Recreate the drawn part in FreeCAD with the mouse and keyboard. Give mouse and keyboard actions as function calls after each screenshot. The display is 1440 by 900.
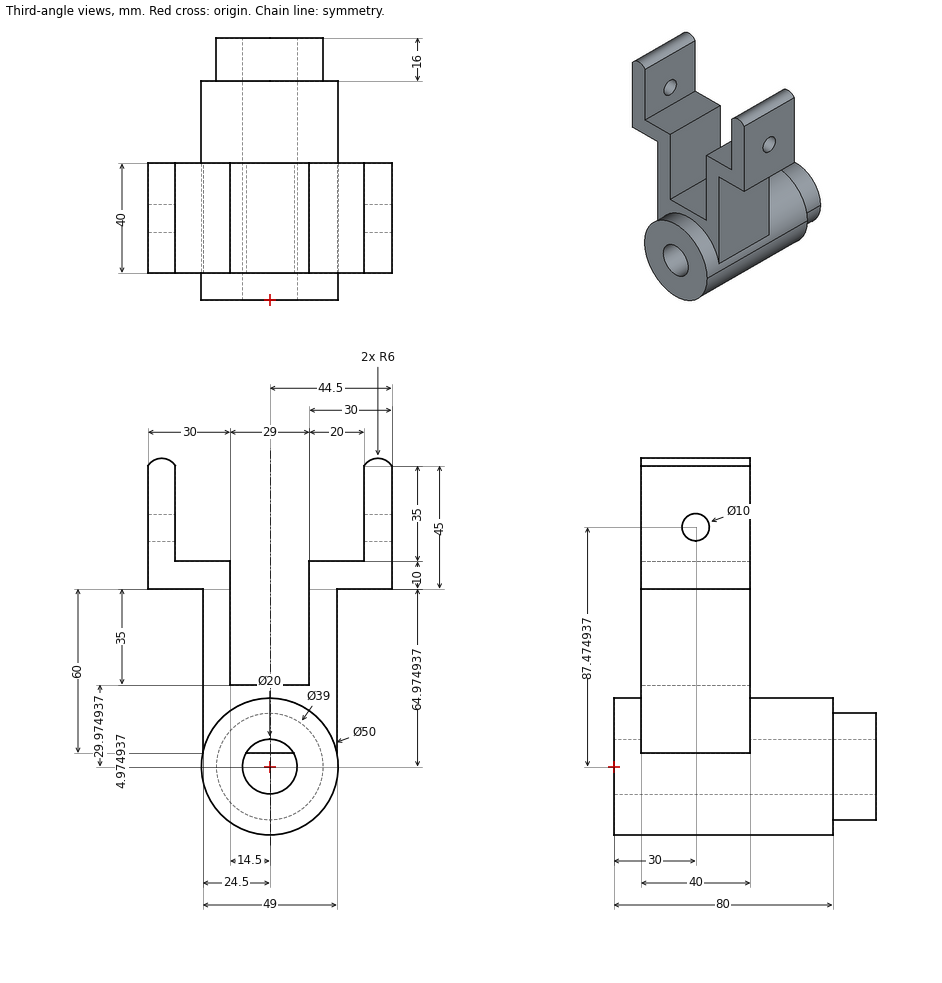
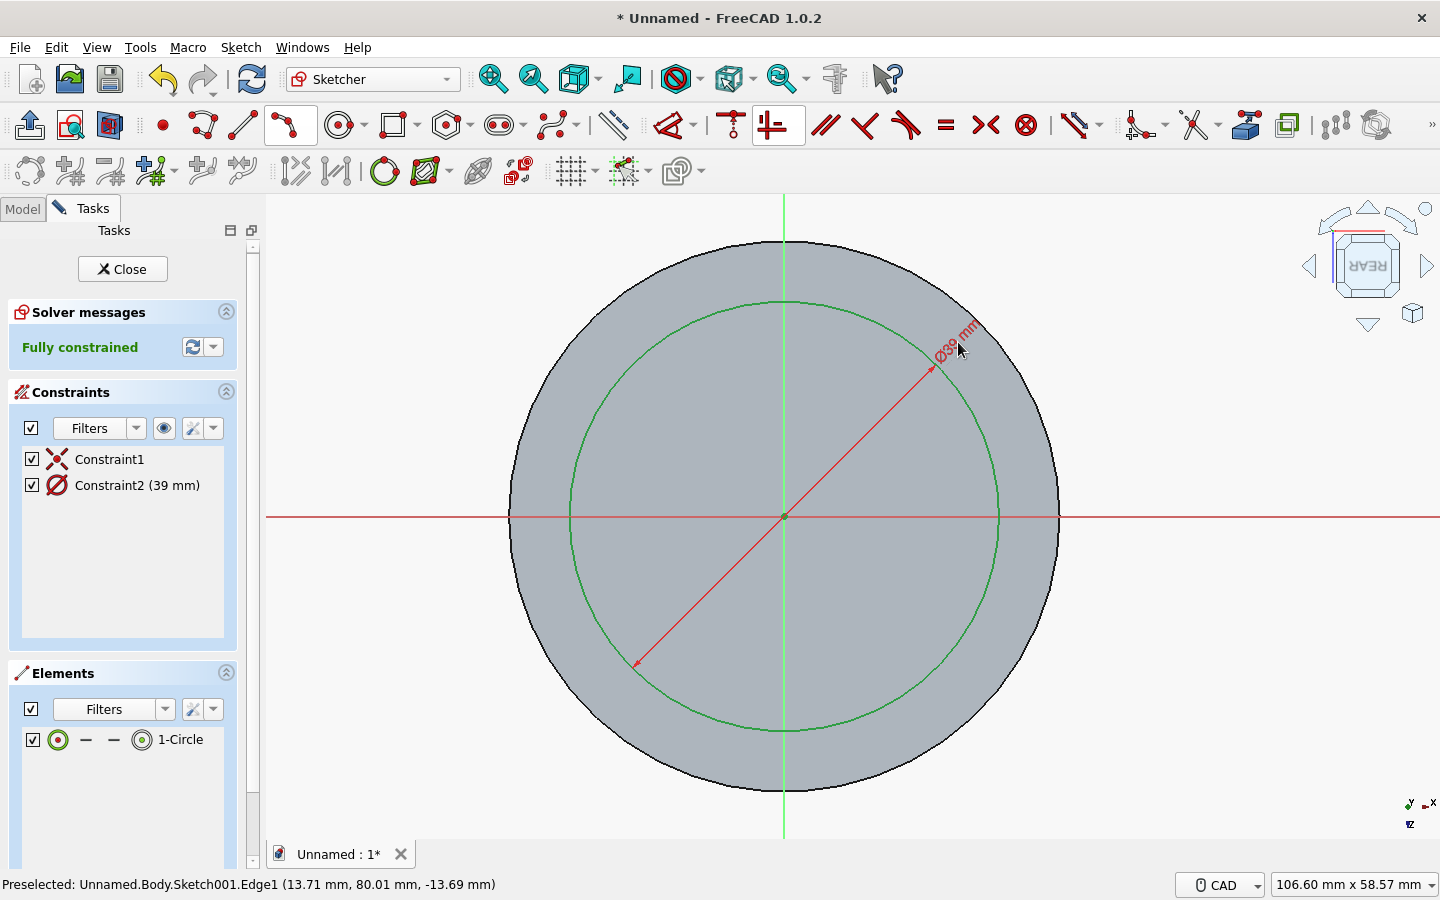
click(123, 269)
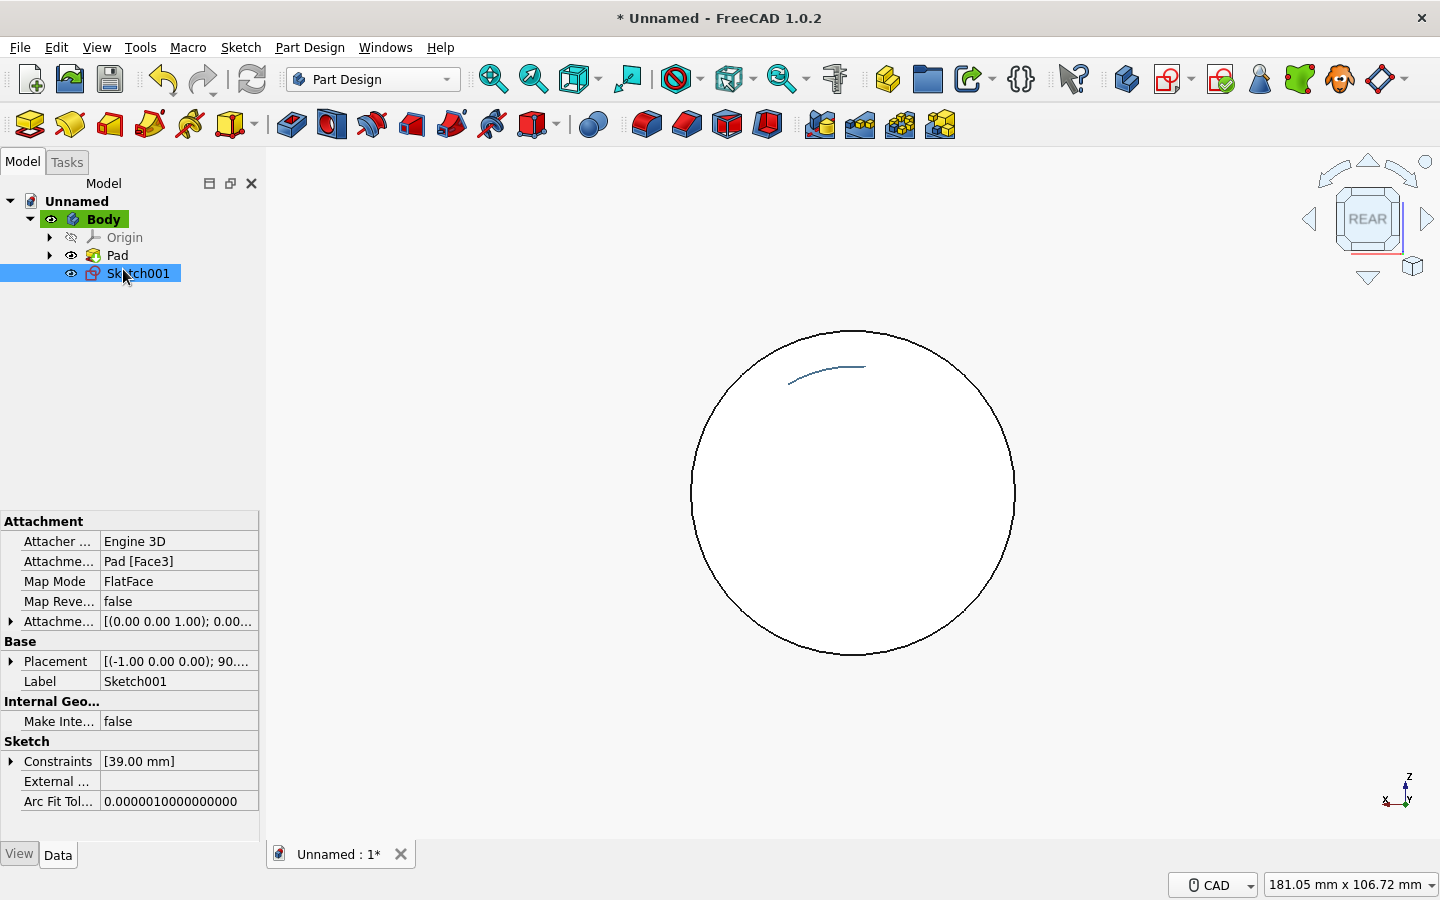
click(30, 124)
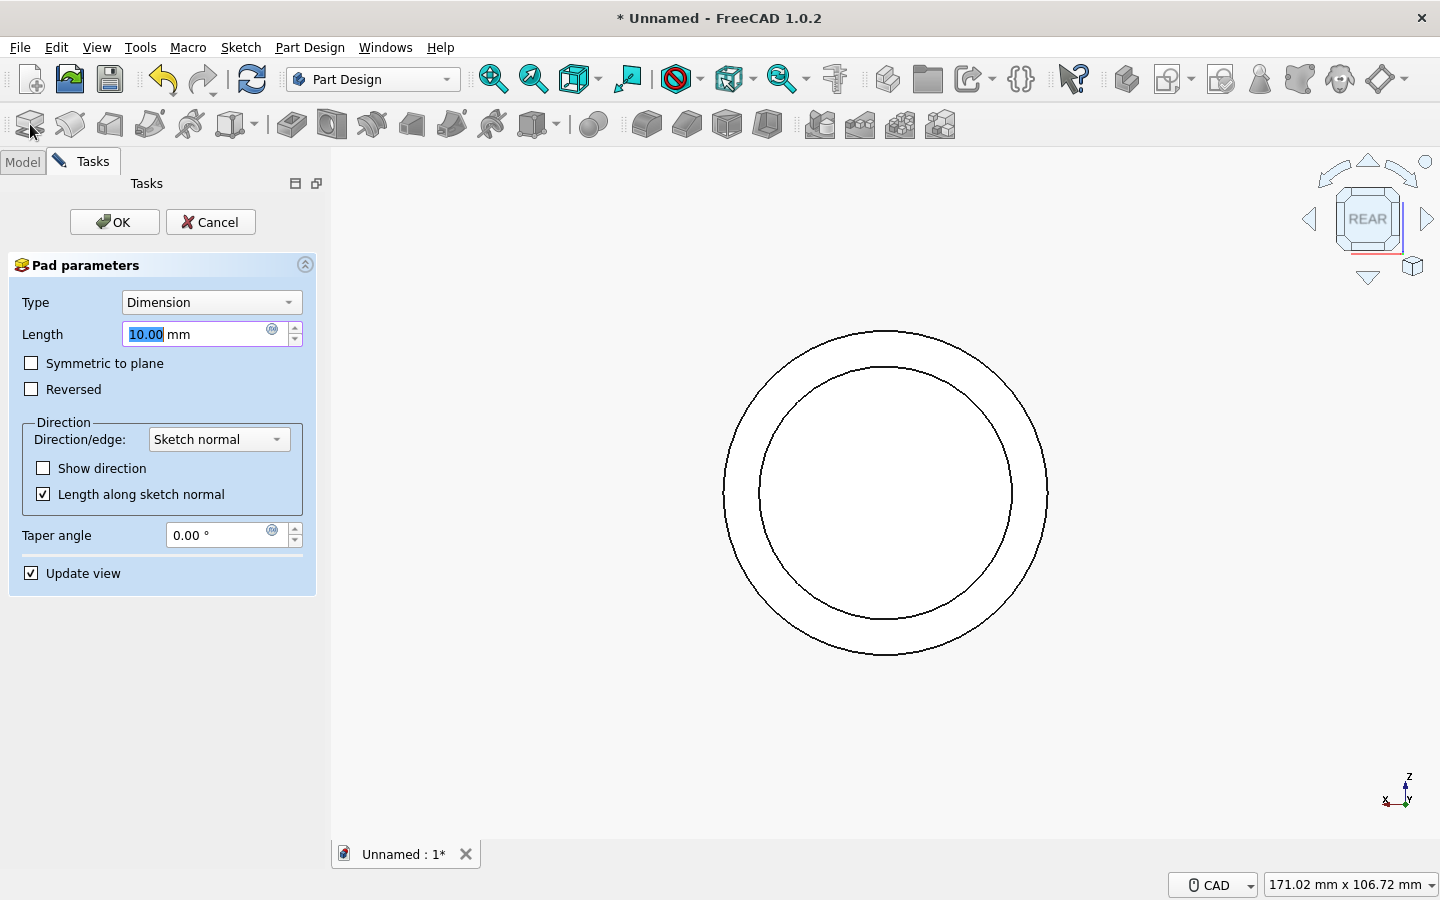
text(16)
key(Tab)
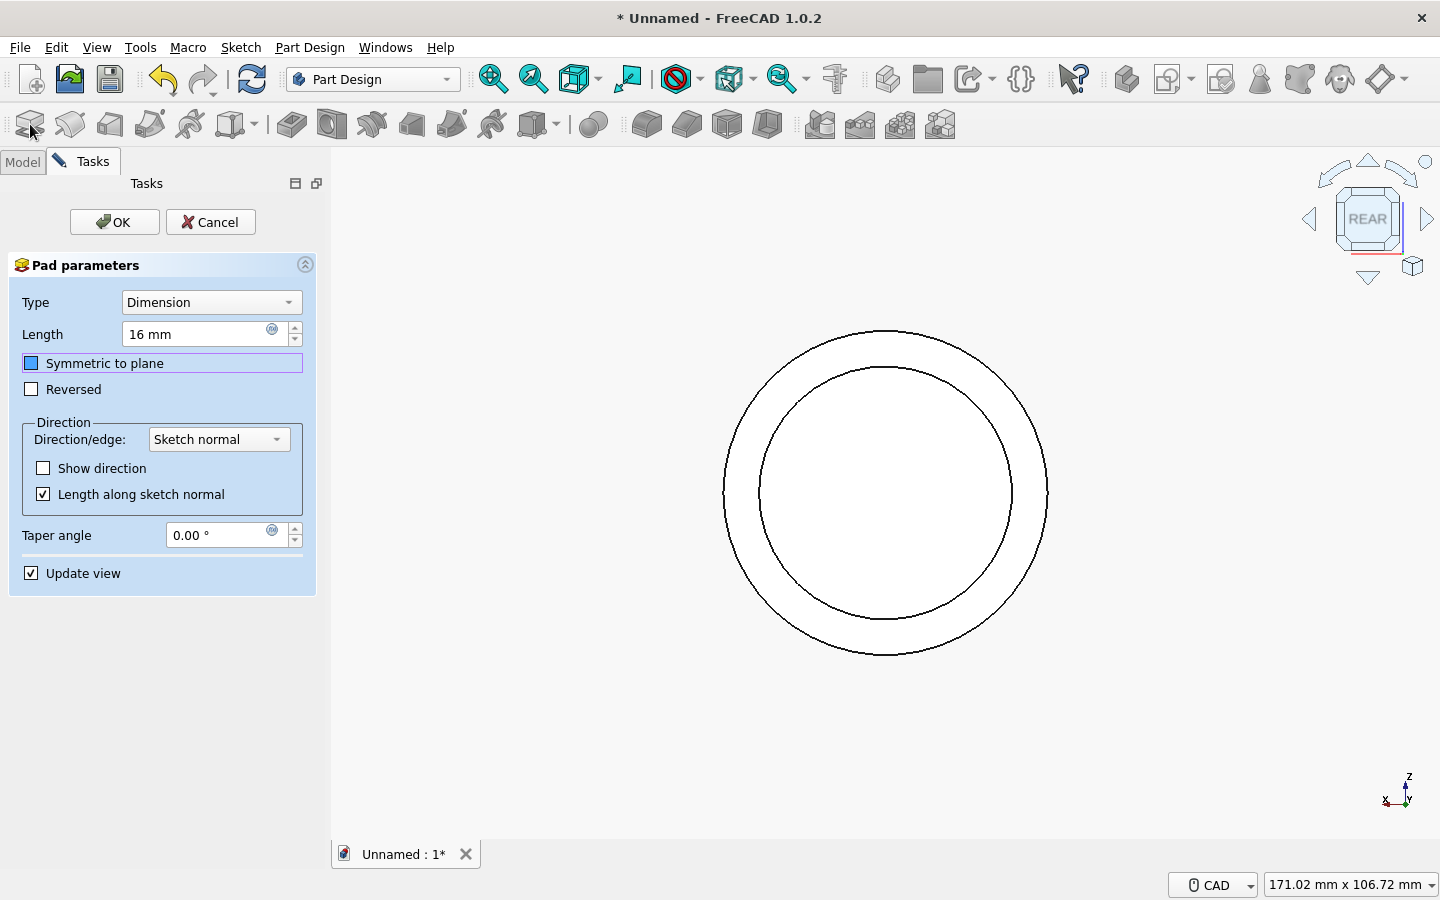
click(115, 222)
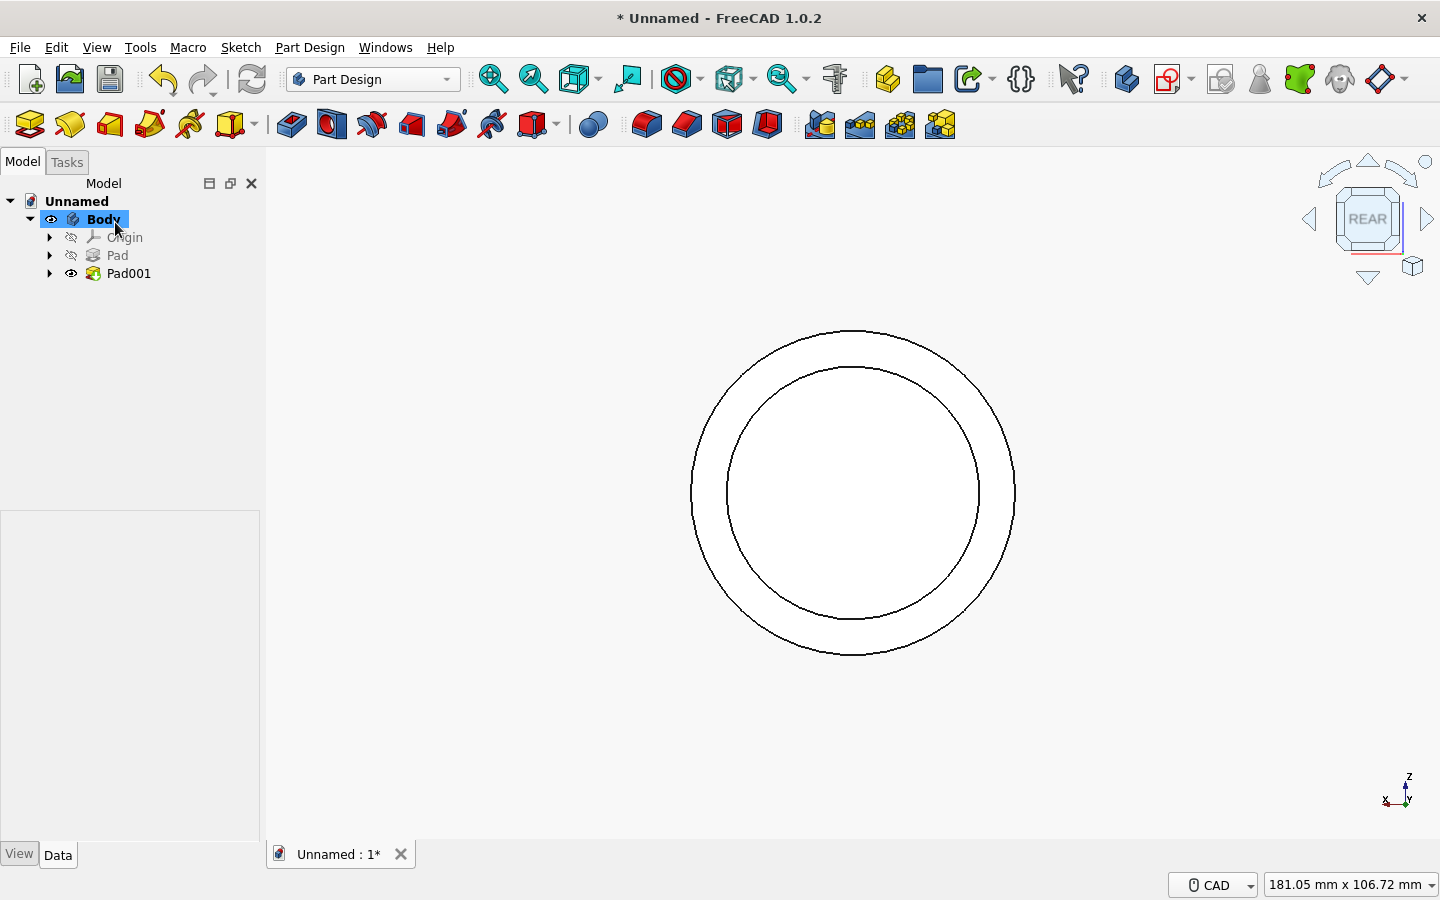
click(853, 492)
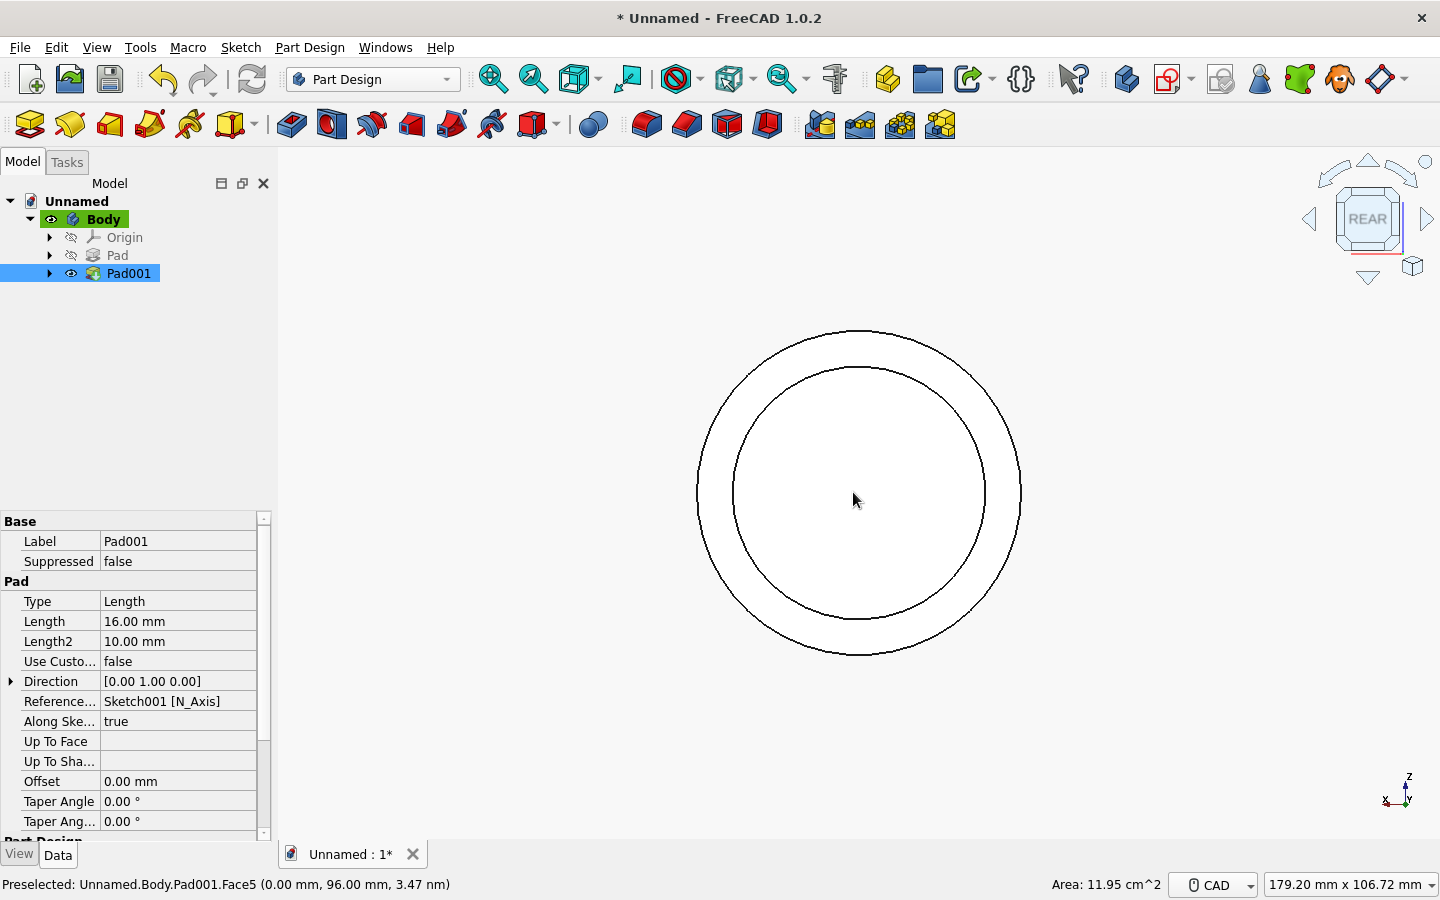
click(1168, 80)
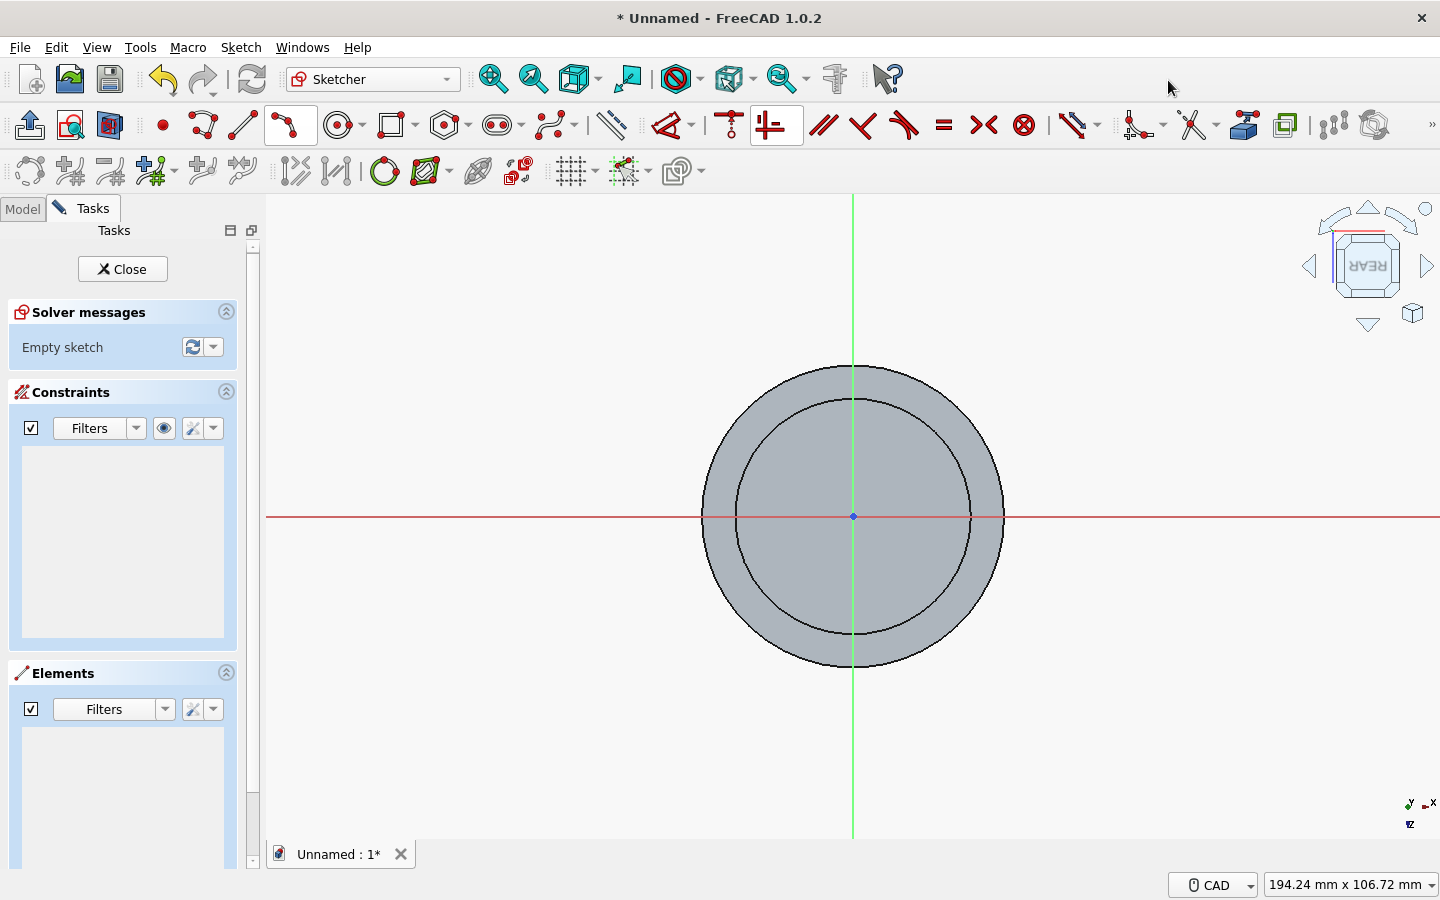
scroll(883, 516, up, 6)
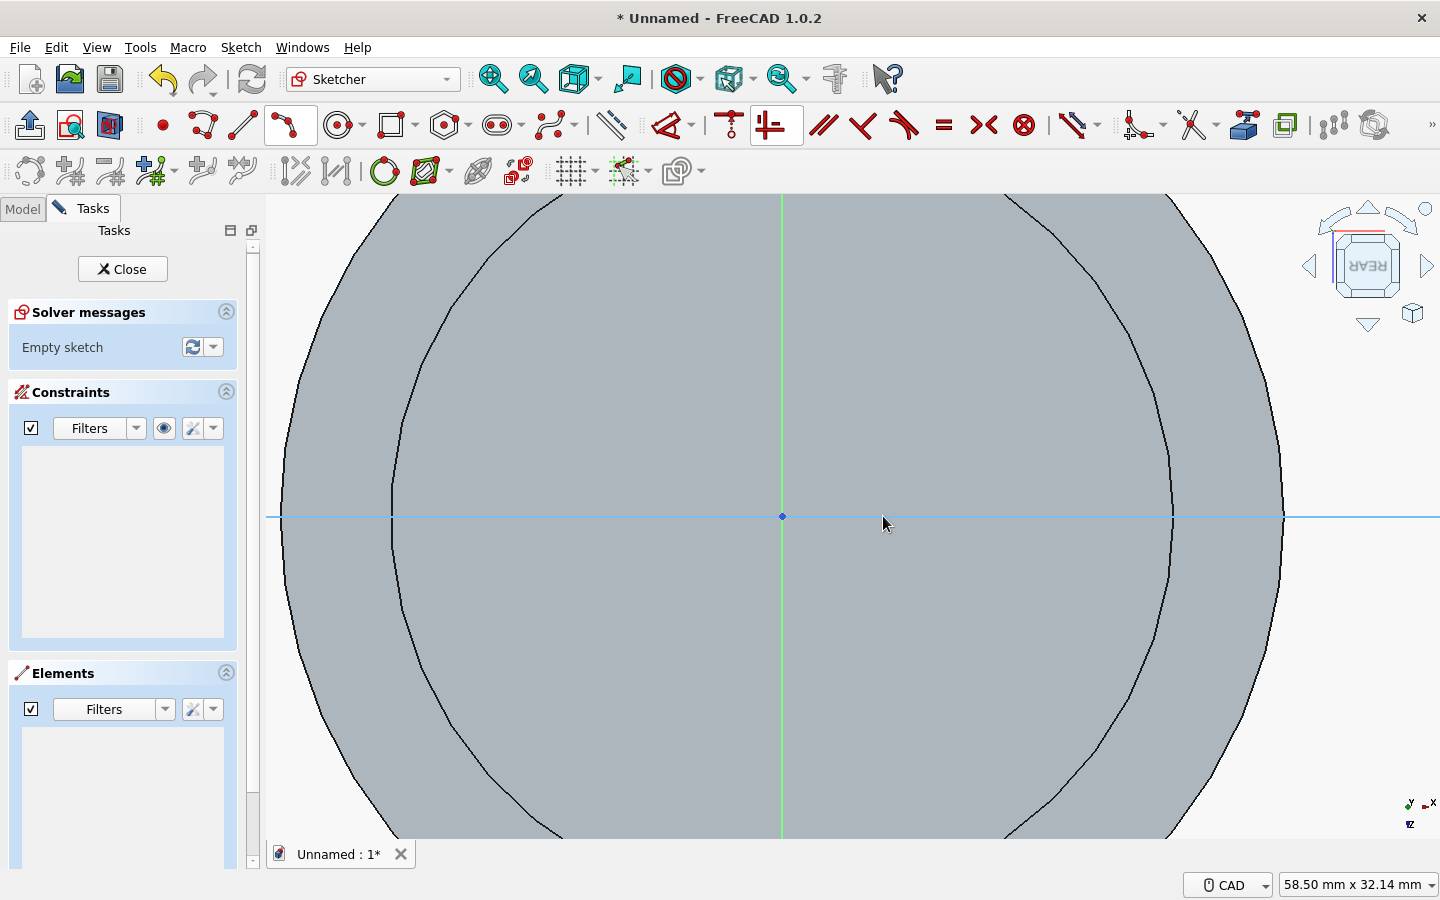
click(338, 126)